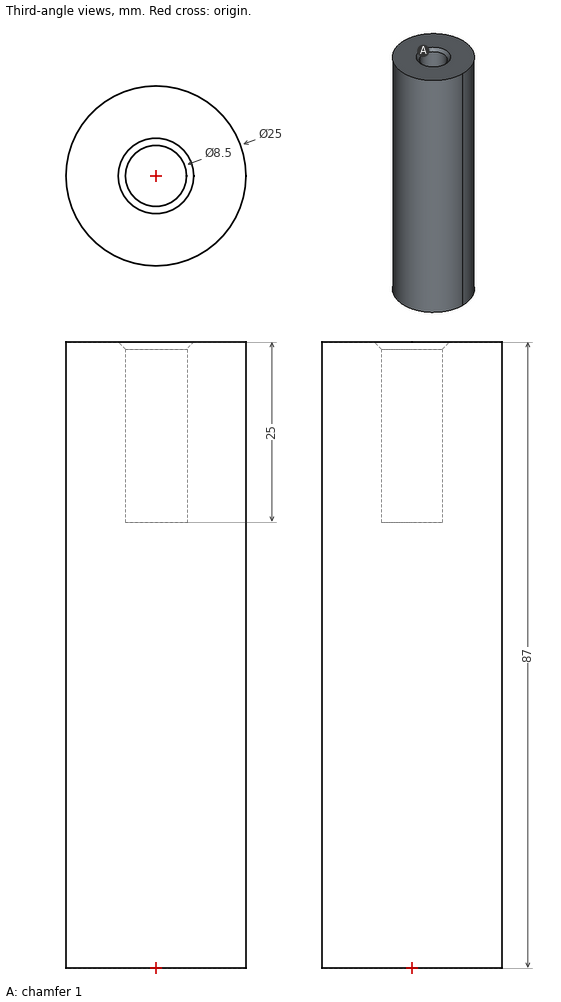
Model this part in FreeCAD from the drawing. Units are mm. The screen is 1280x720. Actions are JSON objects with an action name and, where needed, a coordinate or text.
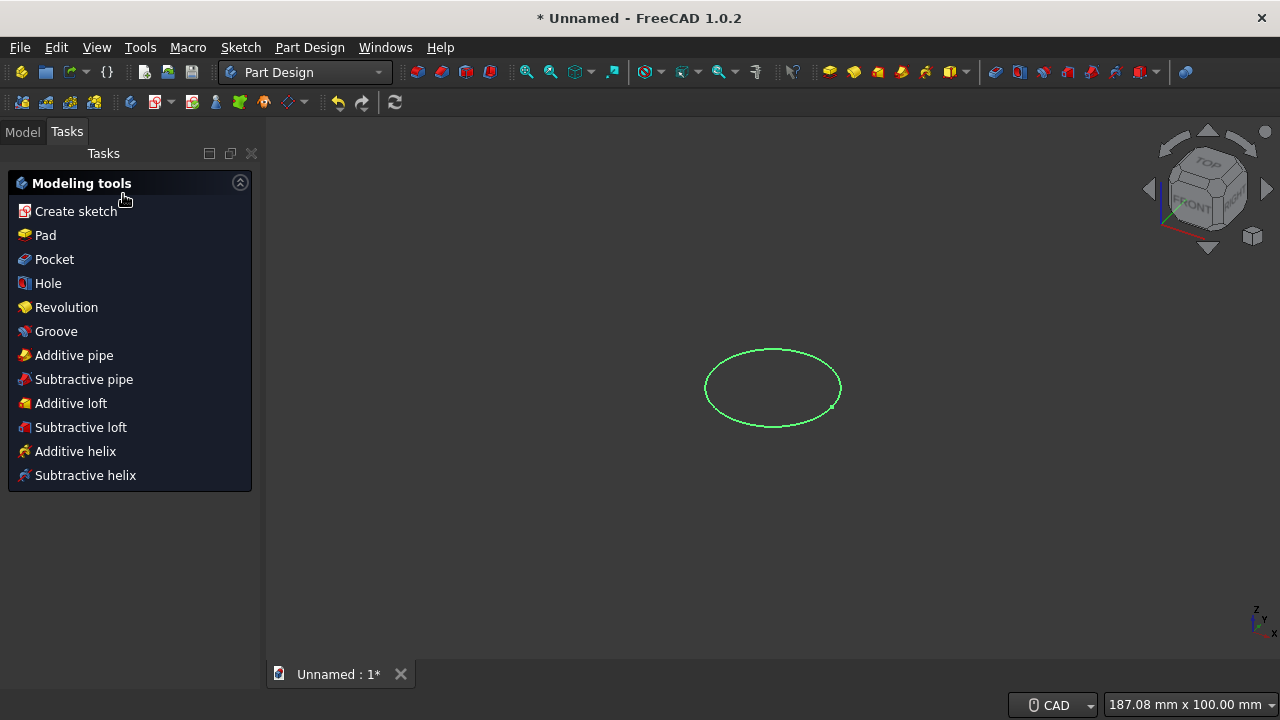
{"action": "left_click", "coordinate": [830, 72]}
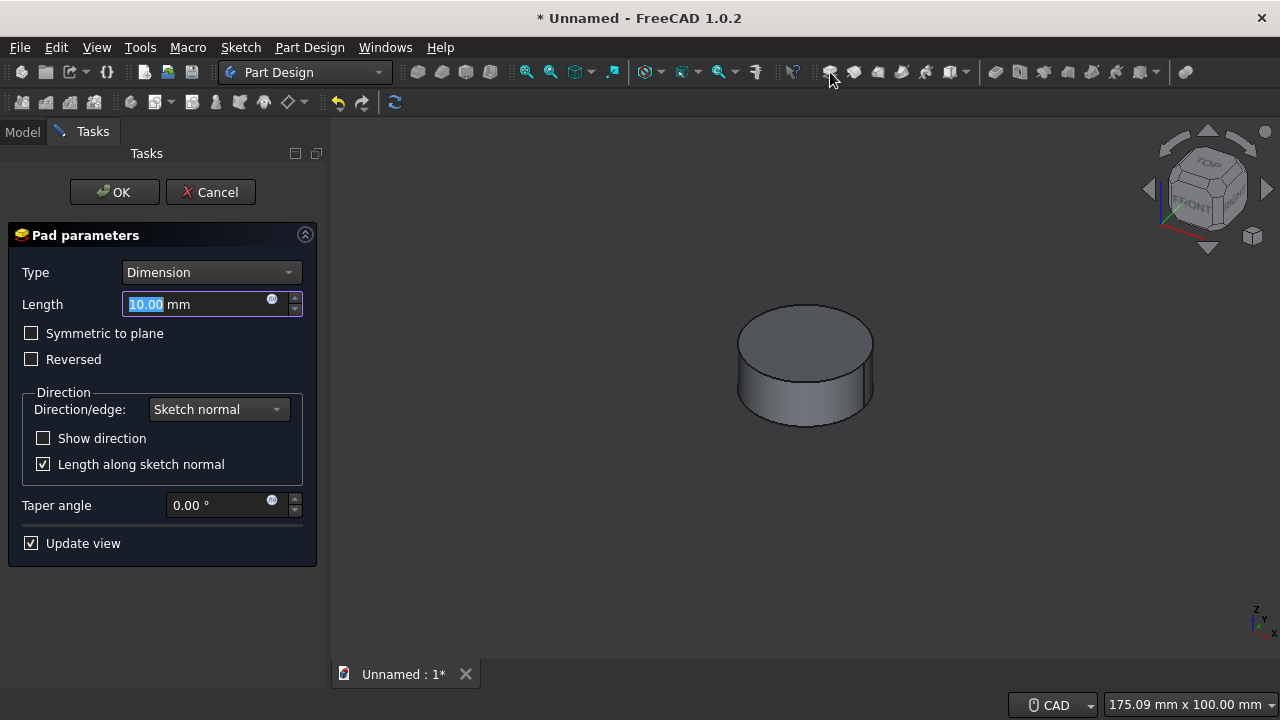
{"action": "type", "text": "87"}
{"action": "key", "text": "Tab"}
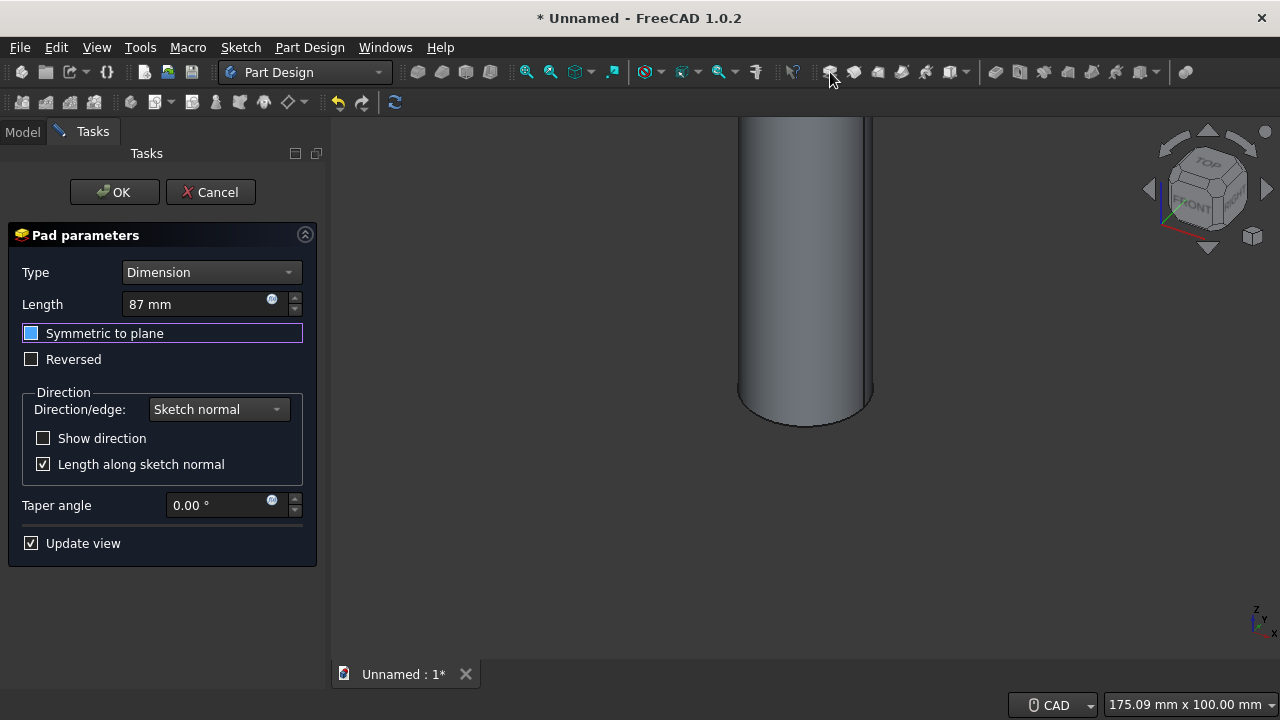
{"action": "left_click", "coordinate": [115, 192]}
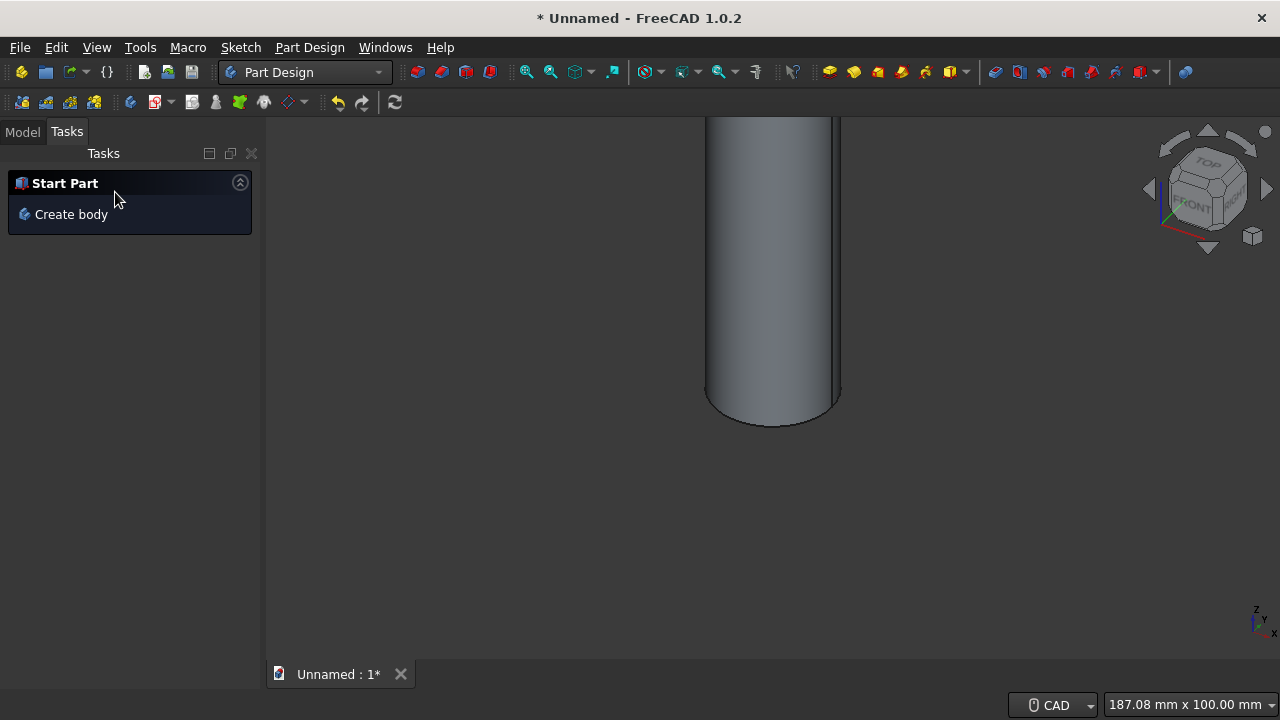
{"action": "key", "text": "v f"}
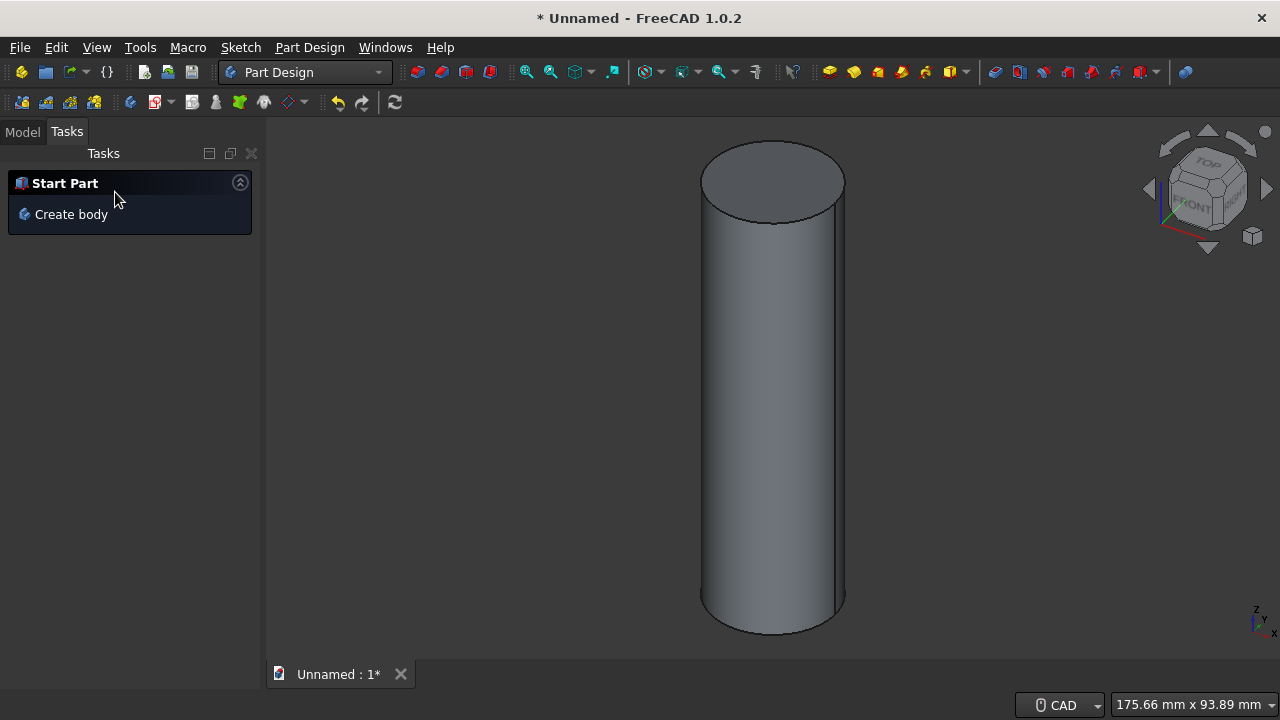
{"action": "left_click", "coordinate": [773, 181]}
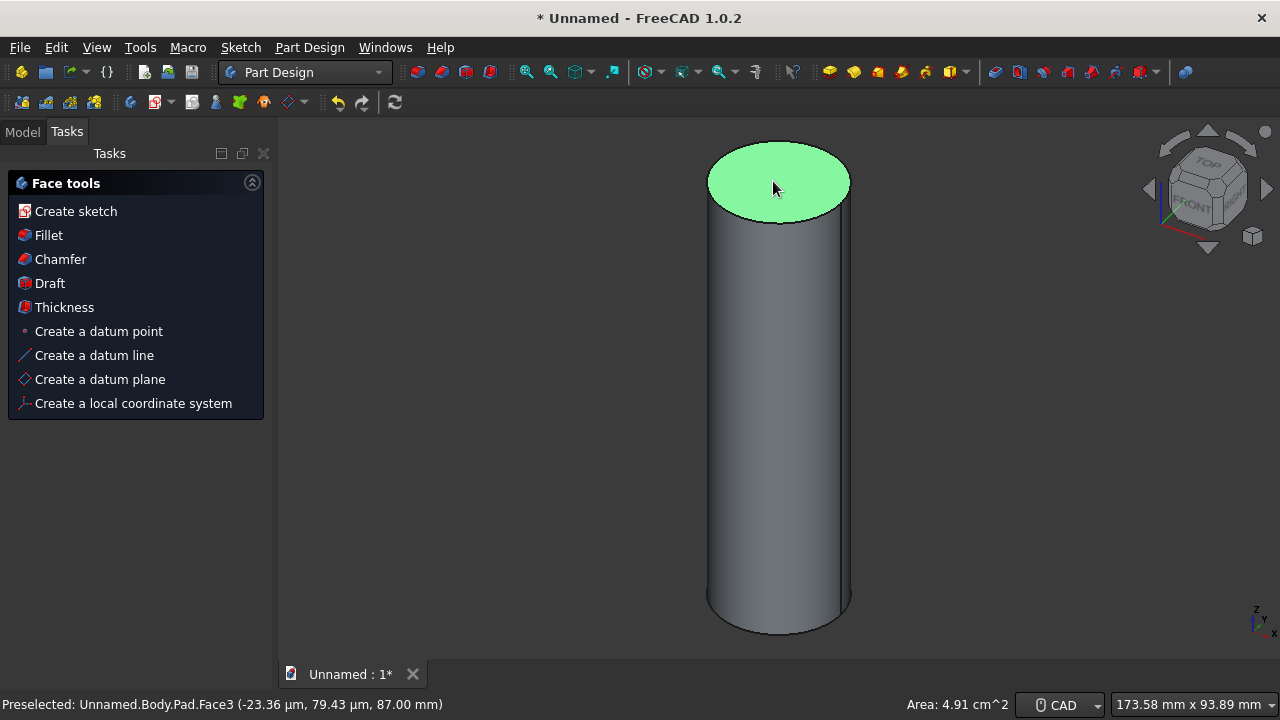
{"action": "left_click", "coordinate": [156, 102]}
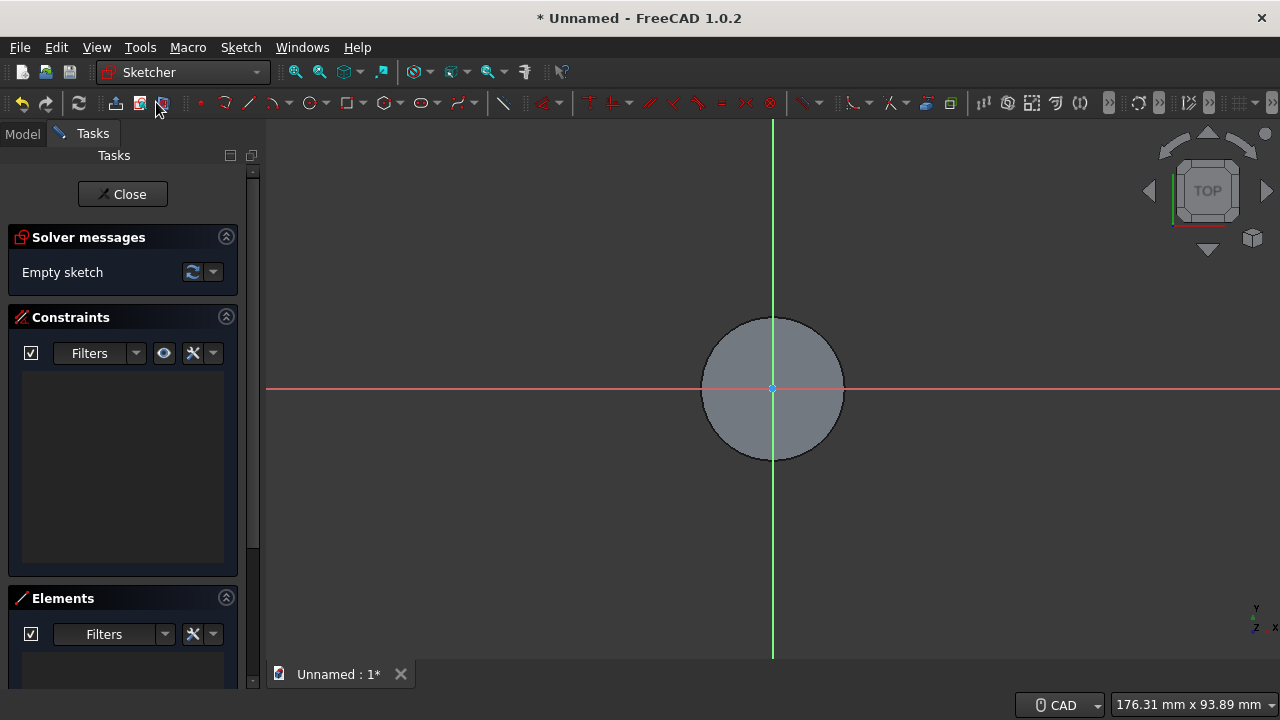
{"action": "scroll", "coordinate": [784, 389], "scroll_direction": "up", "scroll_amount": 10}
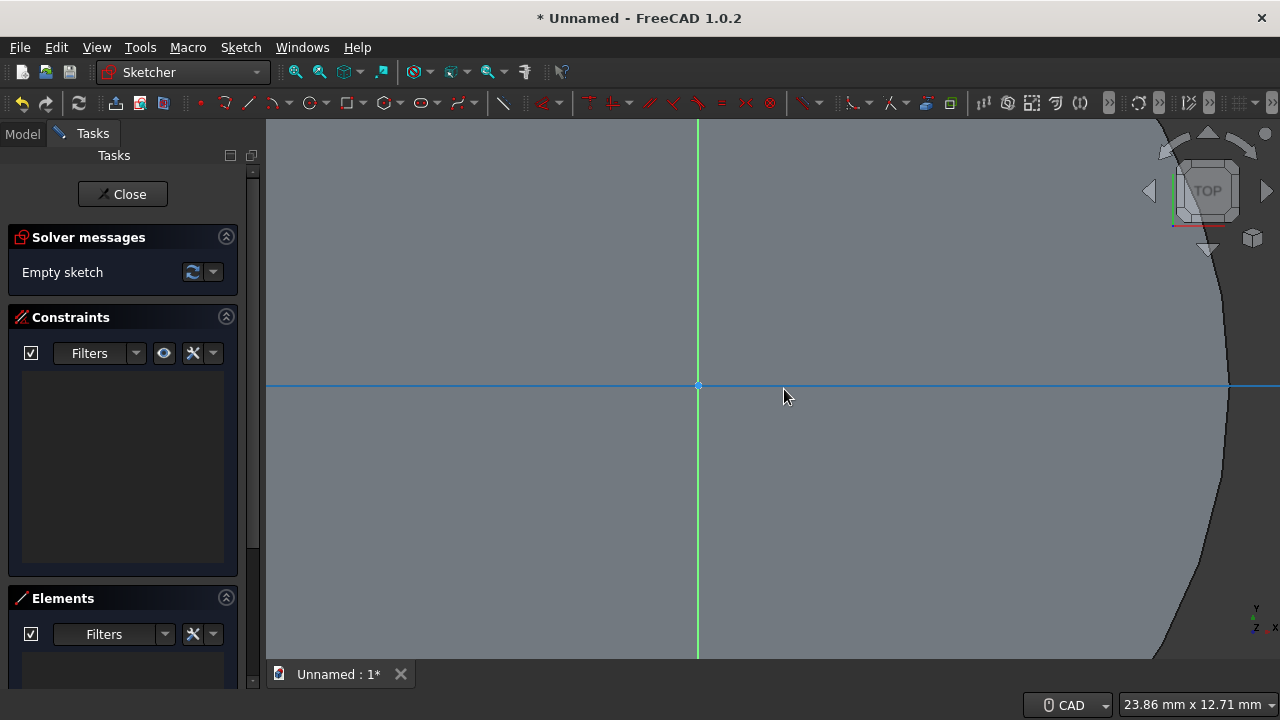
{"action": "left_click", "coordinate": [310, 104]}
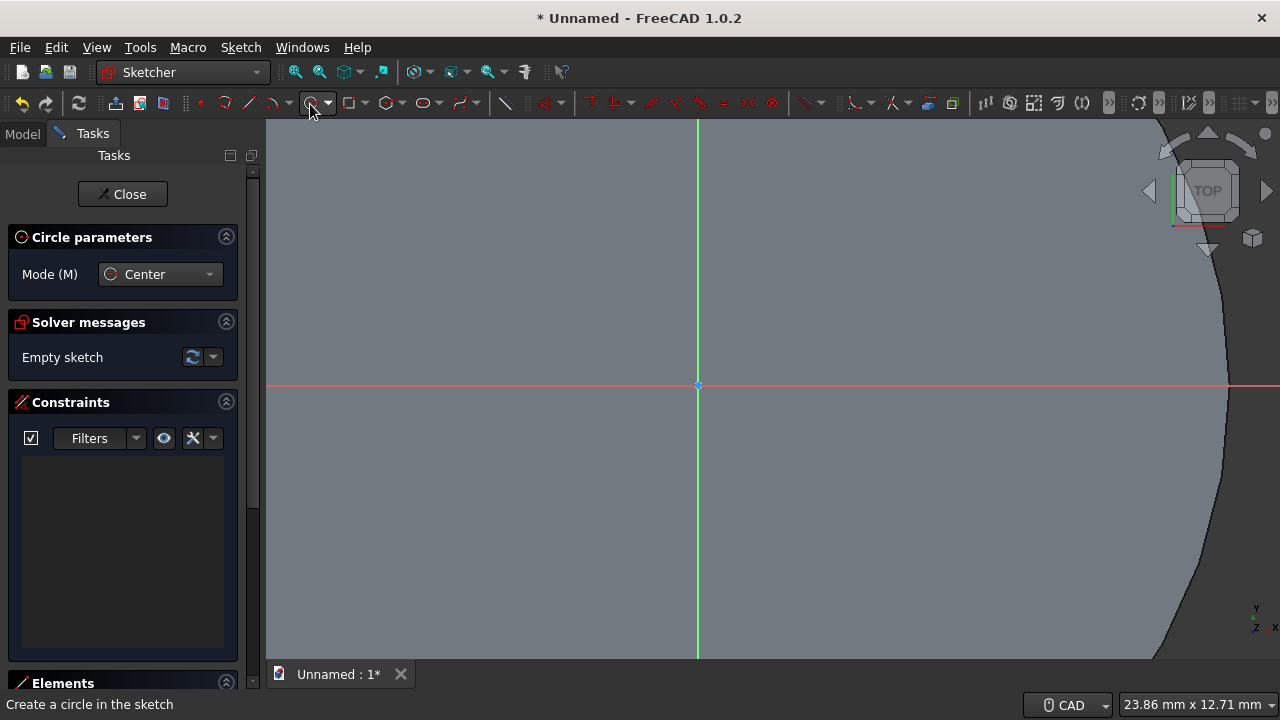
{"action": "left_click", "coordinate": [698, 386]}
{"action": "left_click", "coordinate": [826, 258]}
{"action": "key", "text": "Escape"}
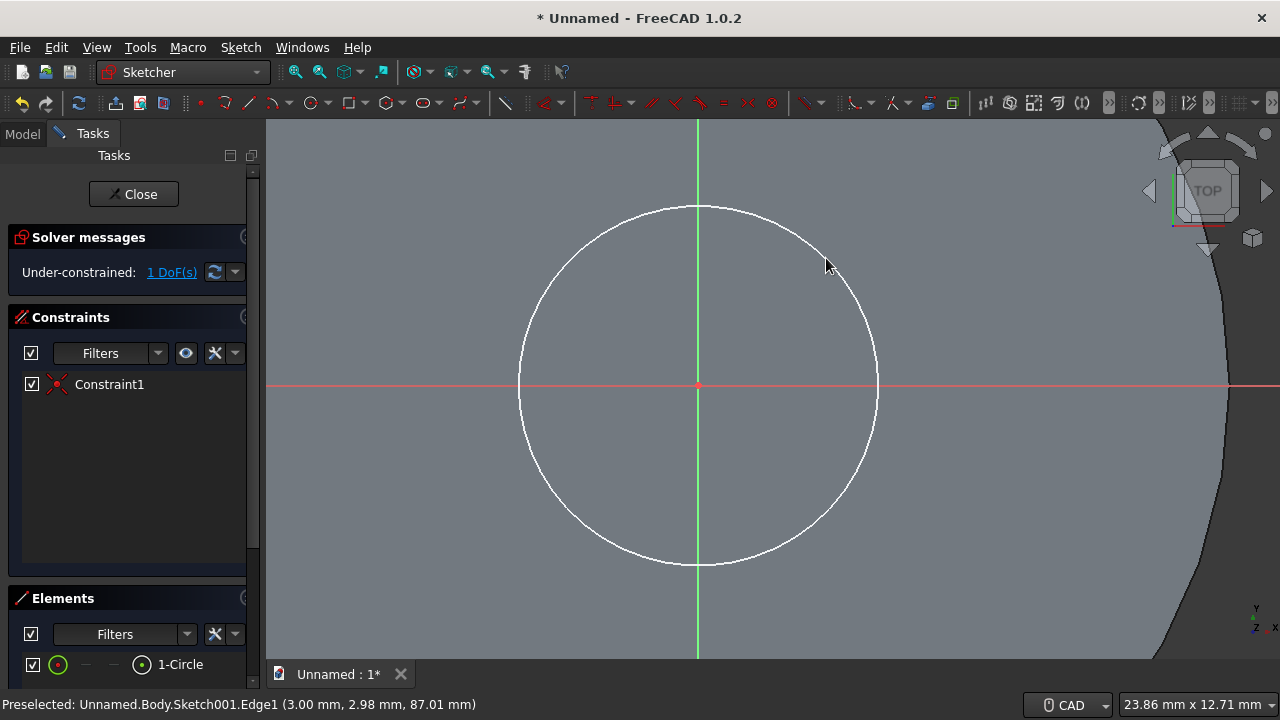
{"action": "left_click", "coordinate": [544, 104]}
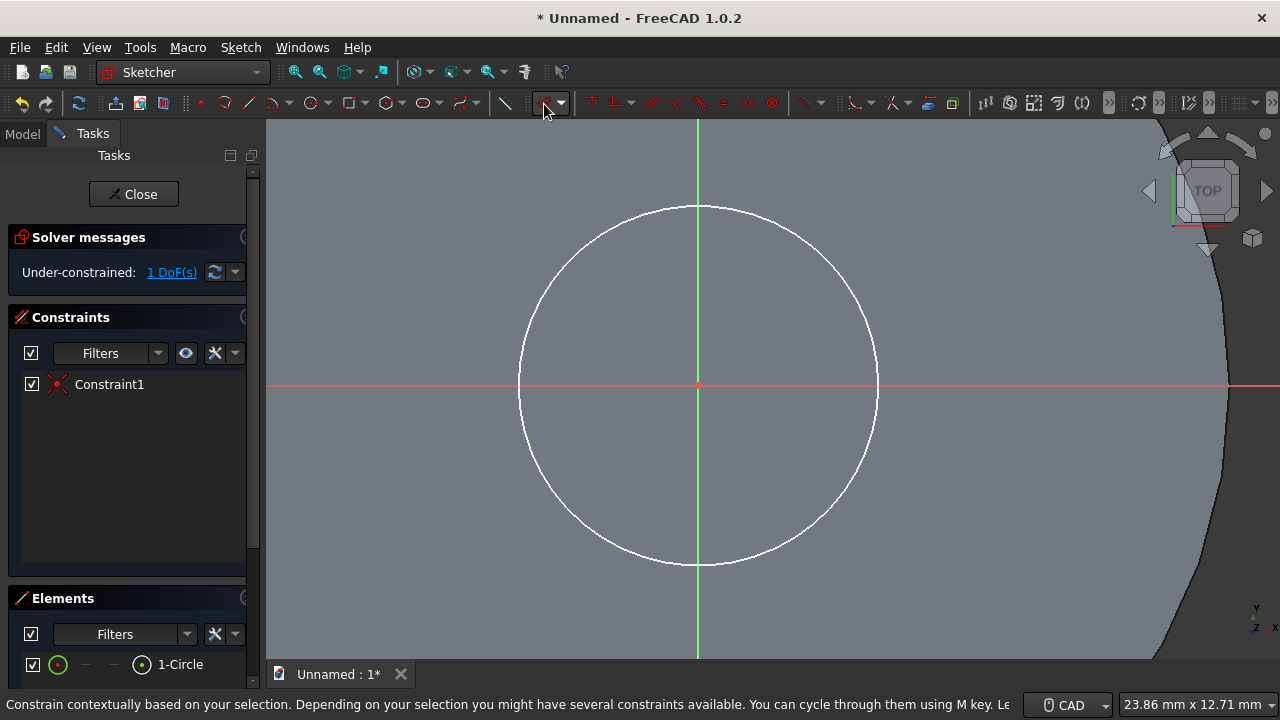
{"action": "left_click", "coordinate": [825, 258]}
{"action": "left_click", "coordinate": [848, 235]}